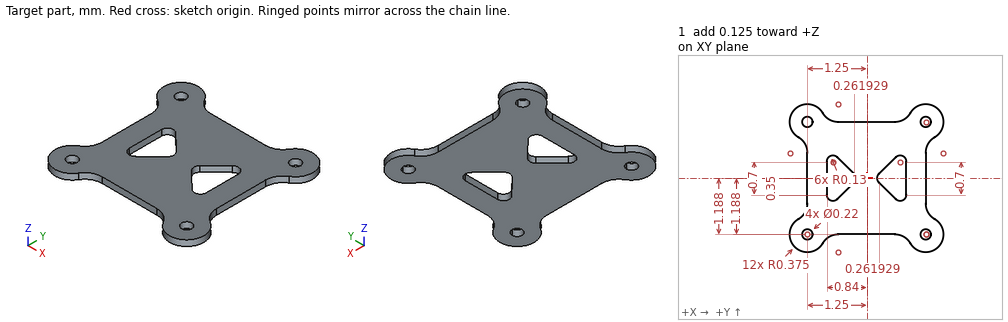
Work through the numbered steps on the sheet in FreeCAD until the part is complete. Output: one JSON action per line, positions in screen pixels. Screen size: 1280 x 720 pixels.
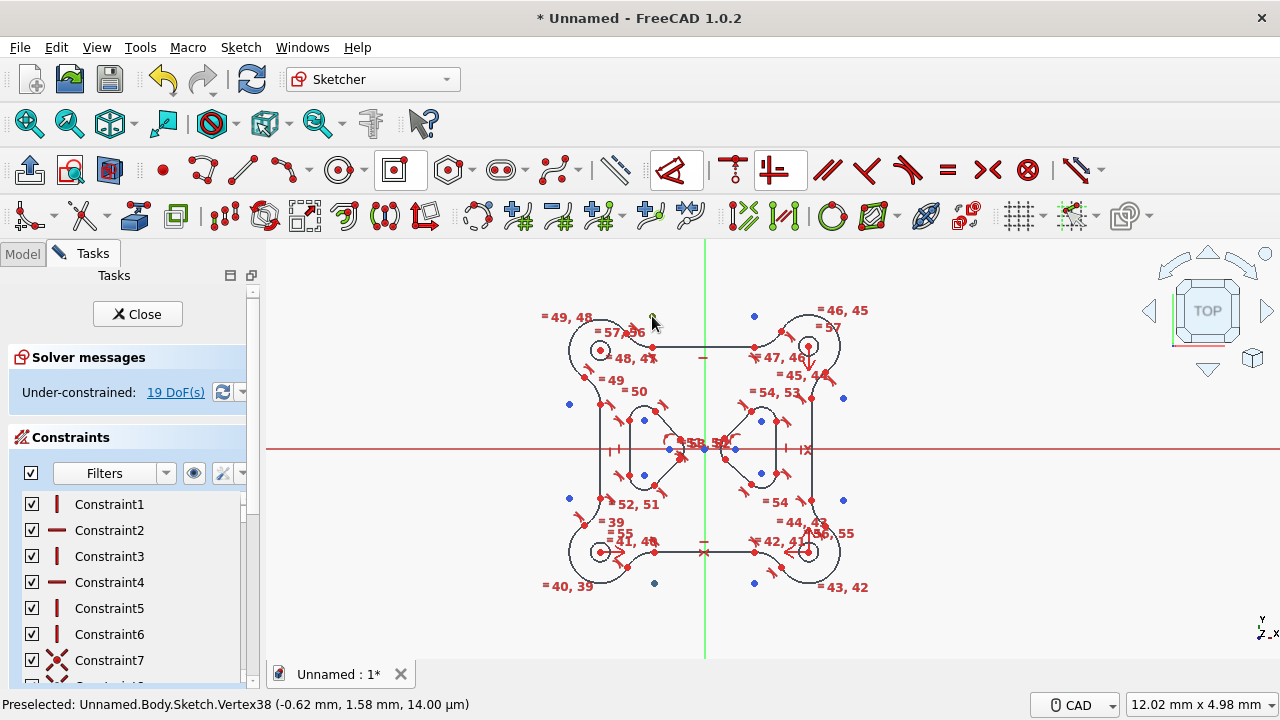
{"action": "left_click", "coordinate": [353, 449]}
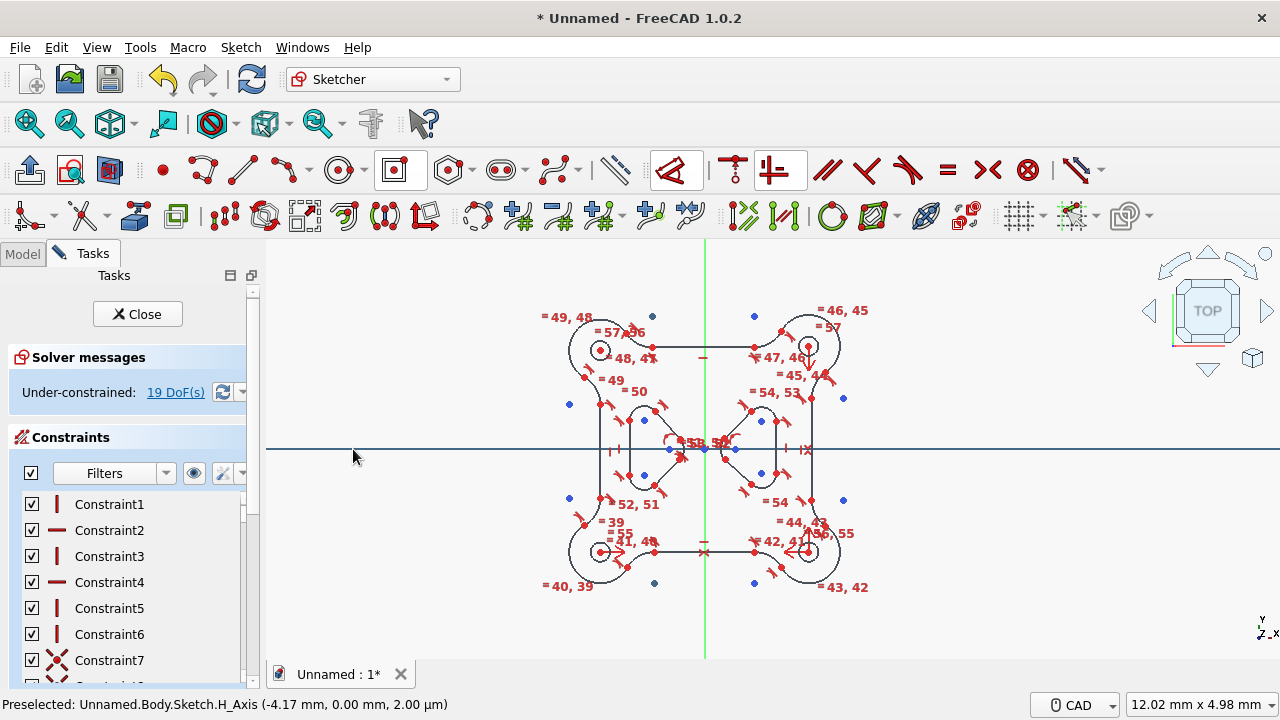
{"action": "left_click", "coordinate": [988, 170]}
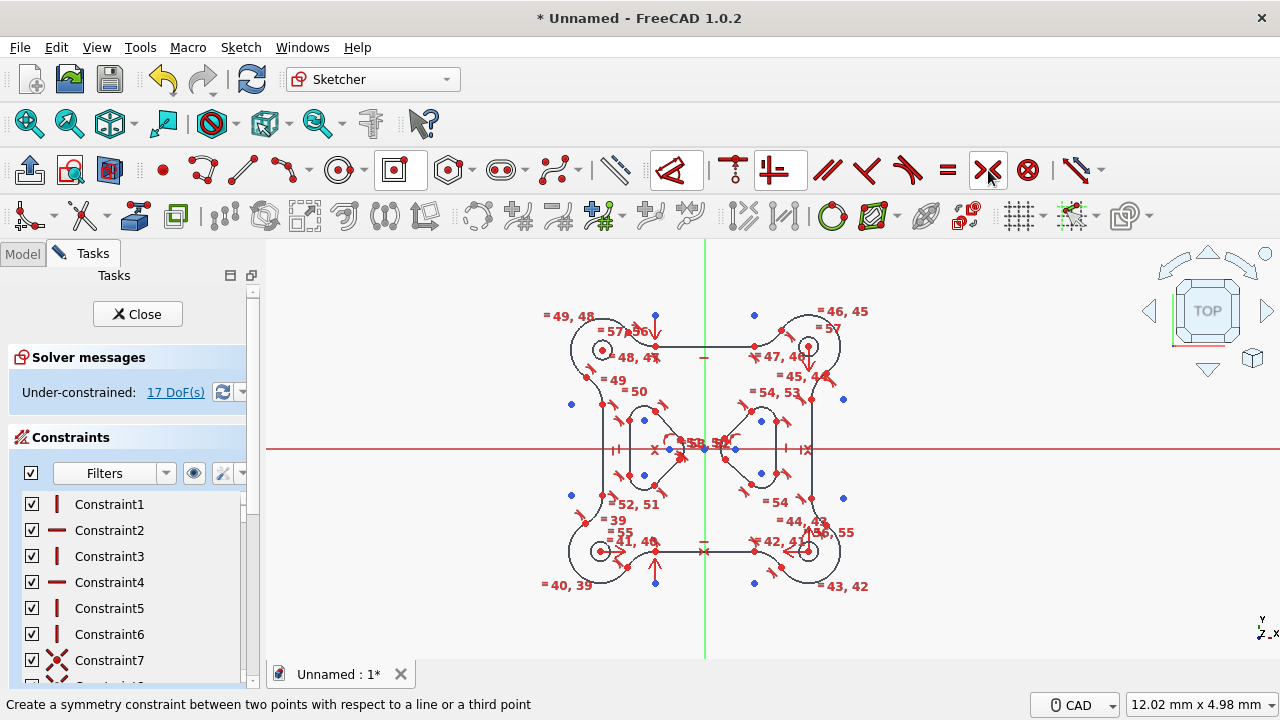
{"action": "left_click", "coordinate": [843, 399]}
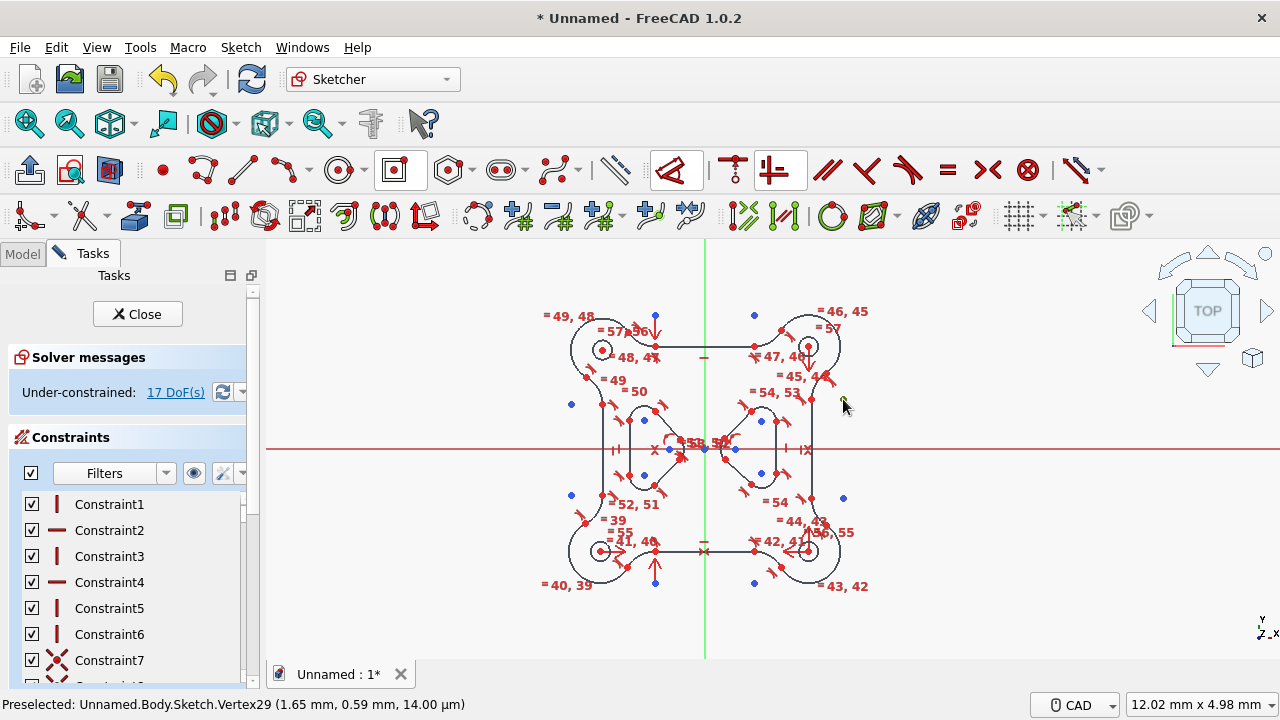
{"action": "left_click", "coordinate": [571, 405]}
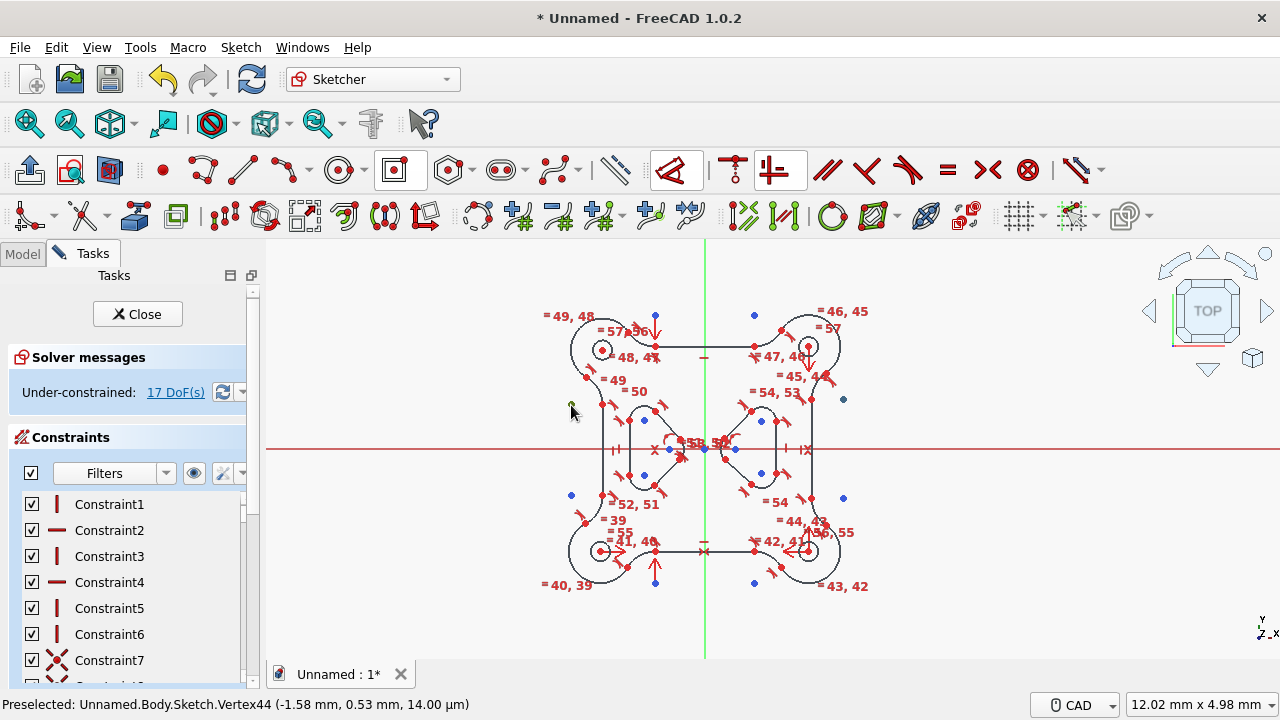
{"action": "left_click", "coordinate": [705, 605]}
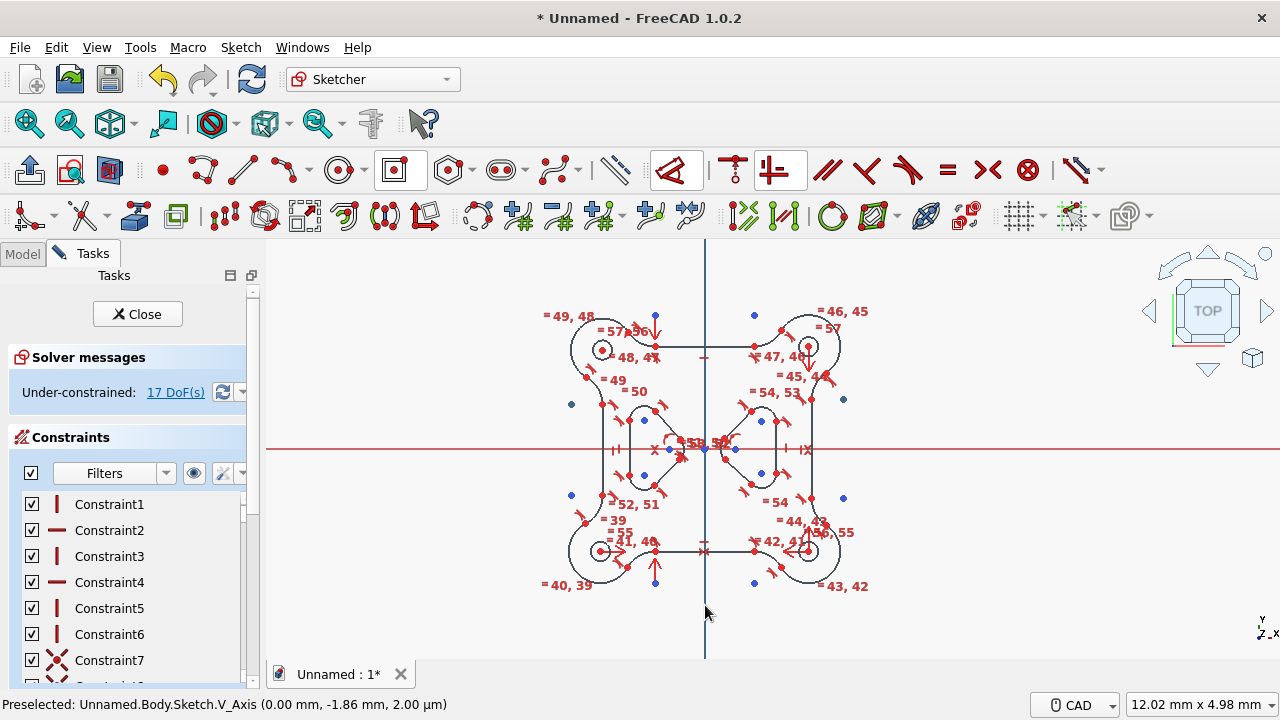
{"action": "left_click", "coordinate": [988, 170]}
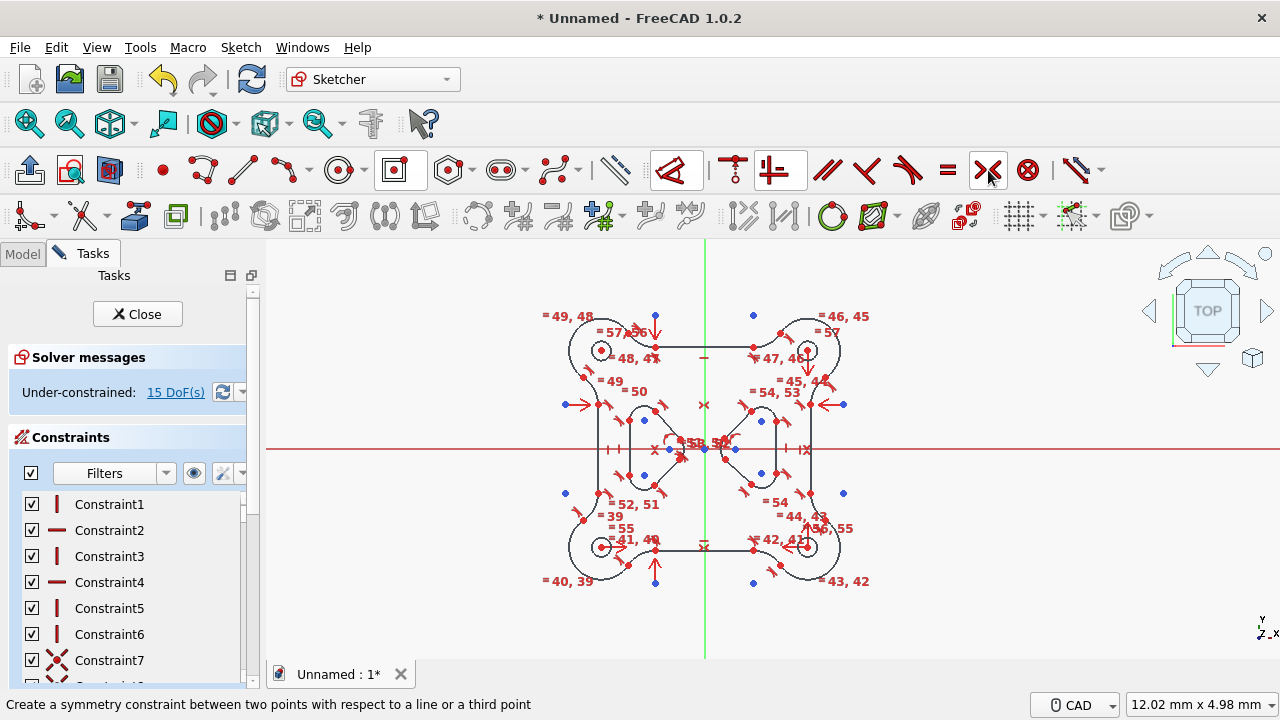
{"action": "left_click", "coordinate": [644, 421]}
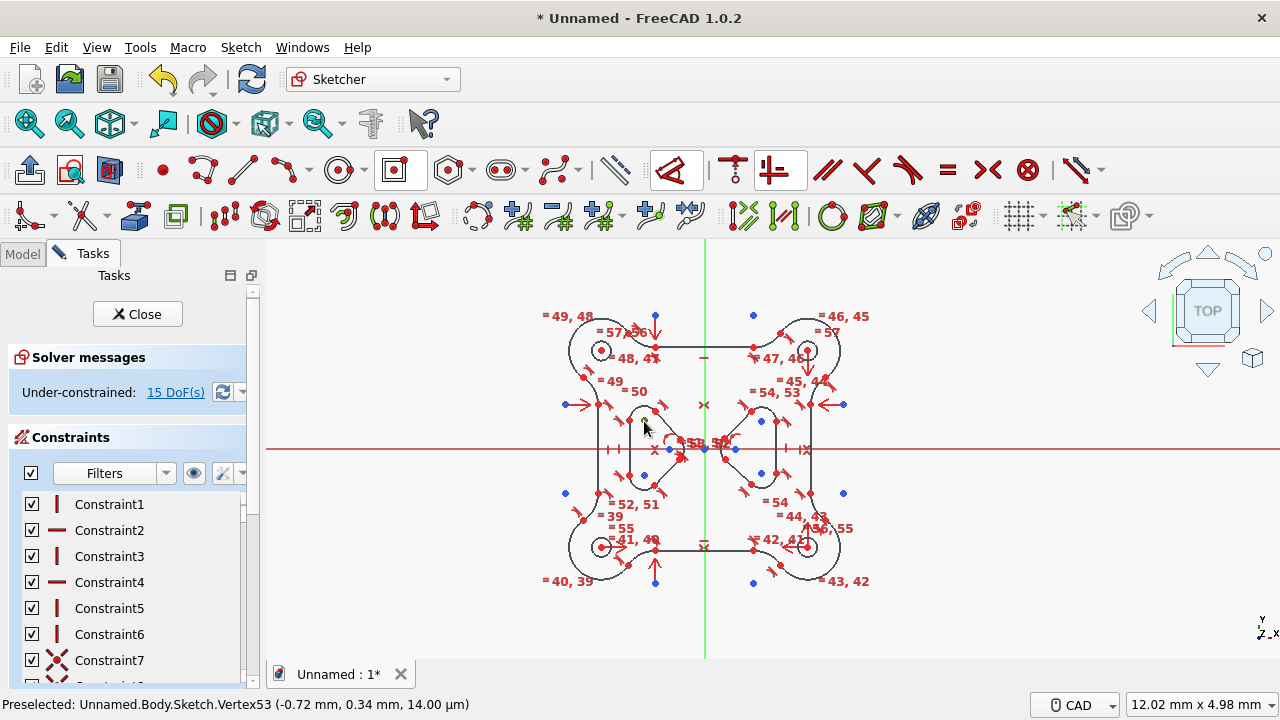
{"action": "left_click", "coordinate": [762, 422]}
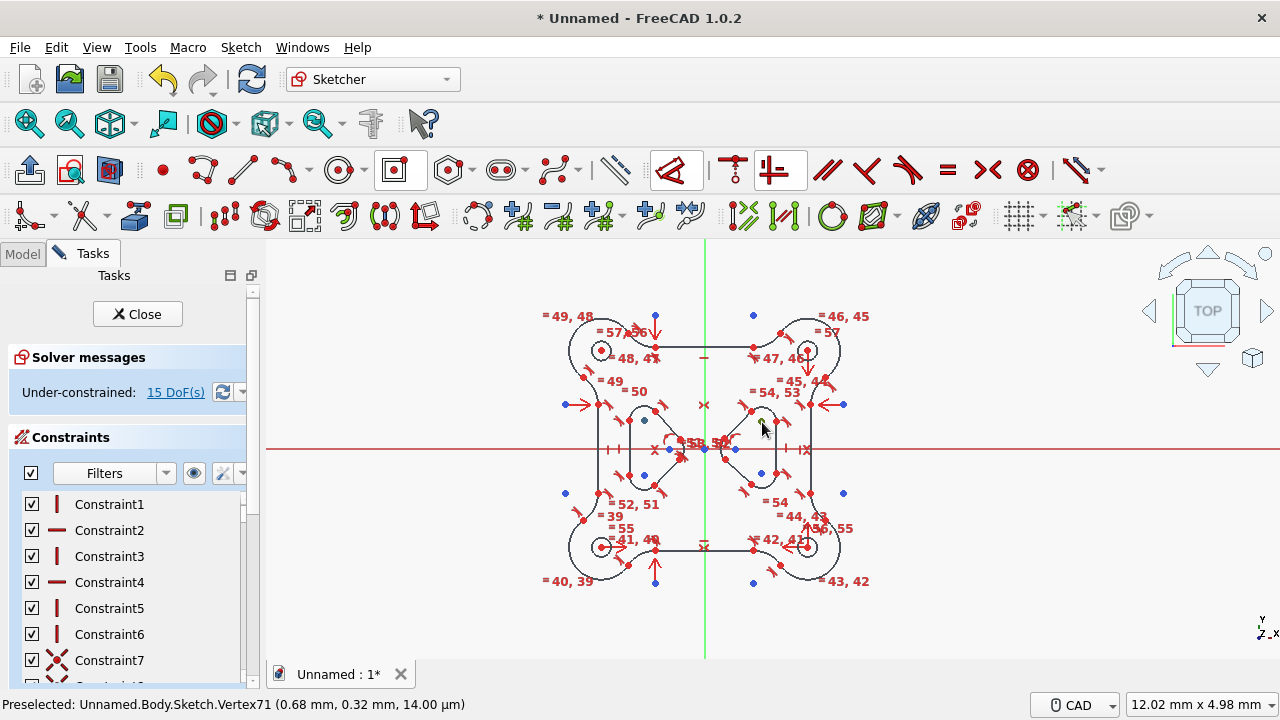
{"action": "left_click", "coordinate": [705, 605]}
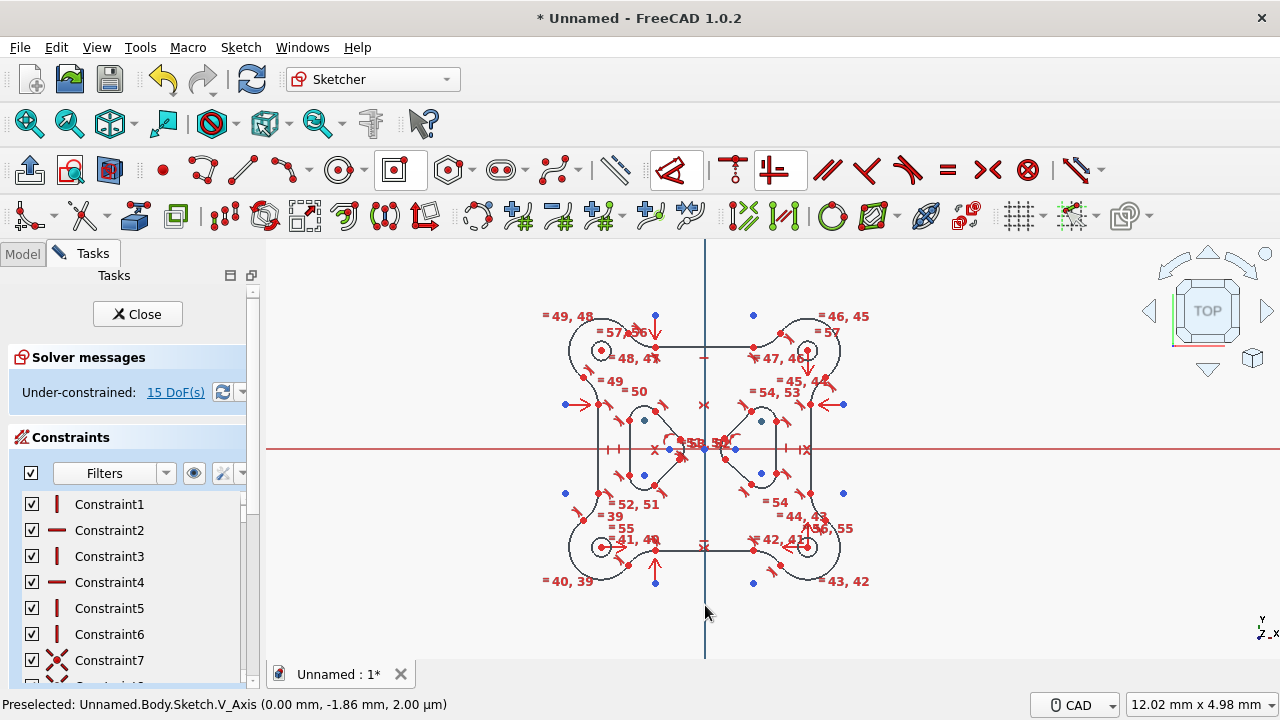
{"action": "left_click", "coordinate": [988, 170]}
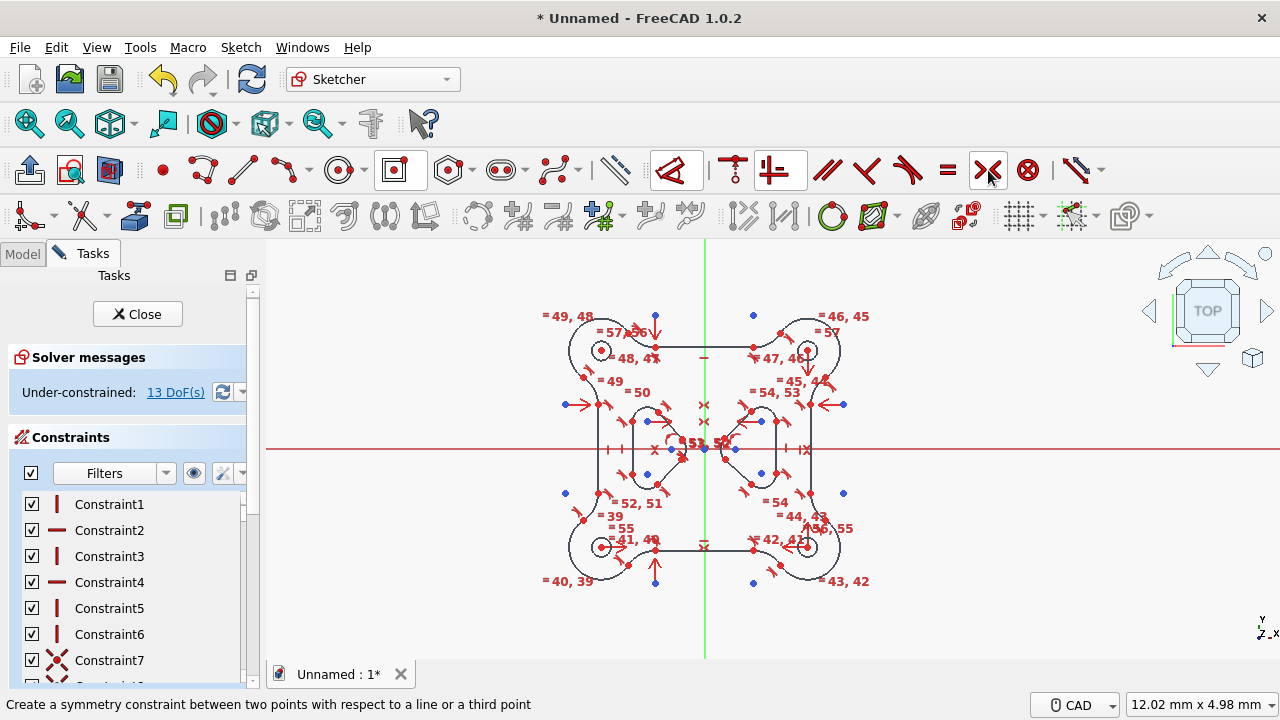
{"action": "left_click", "coordinate": [670, 170]}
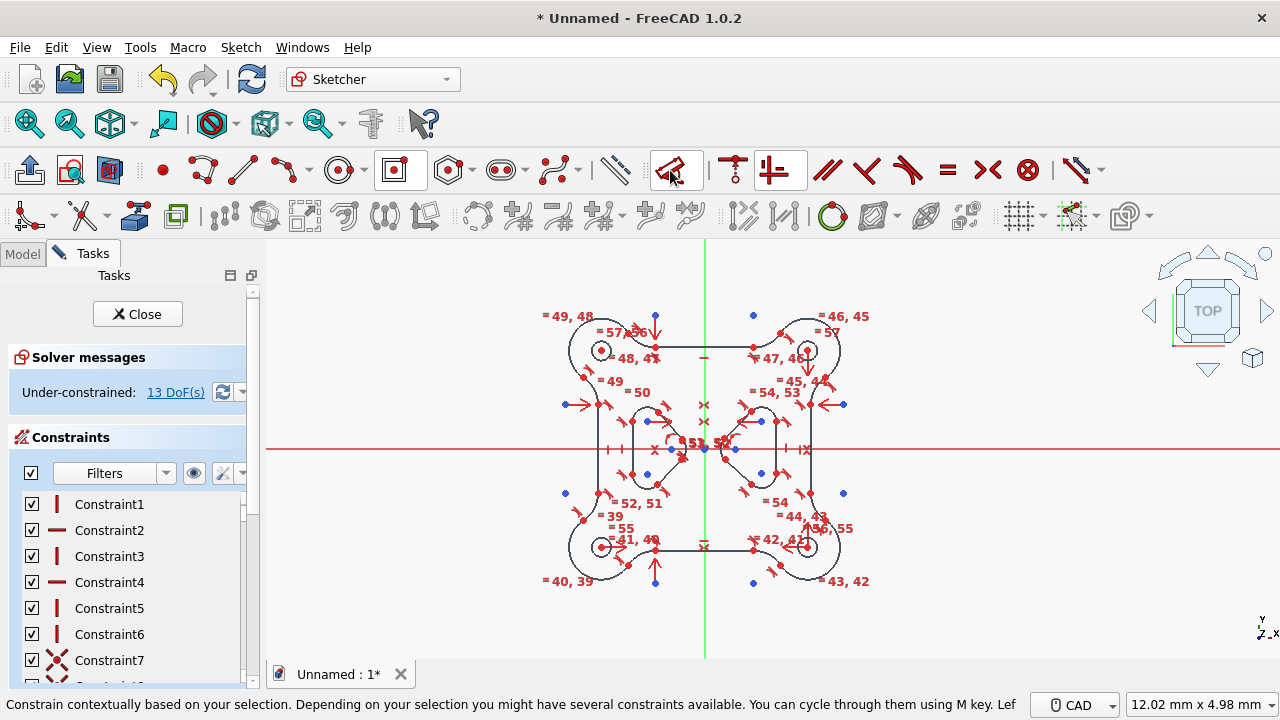
{"action": "scroll", "coordinate": [591, 514], "scroll_direction": "up", "scroll_amount": 2}